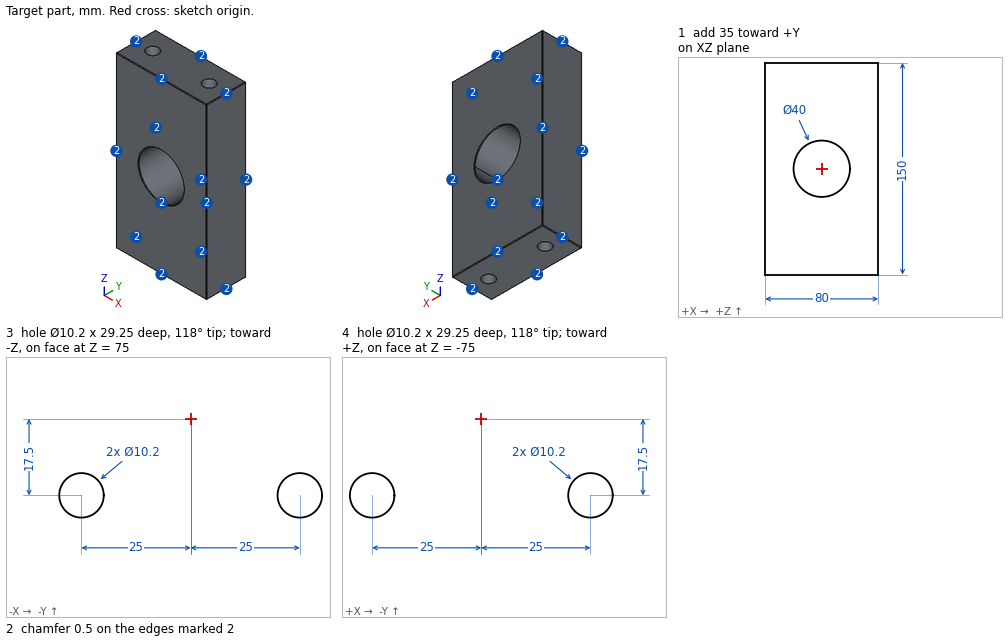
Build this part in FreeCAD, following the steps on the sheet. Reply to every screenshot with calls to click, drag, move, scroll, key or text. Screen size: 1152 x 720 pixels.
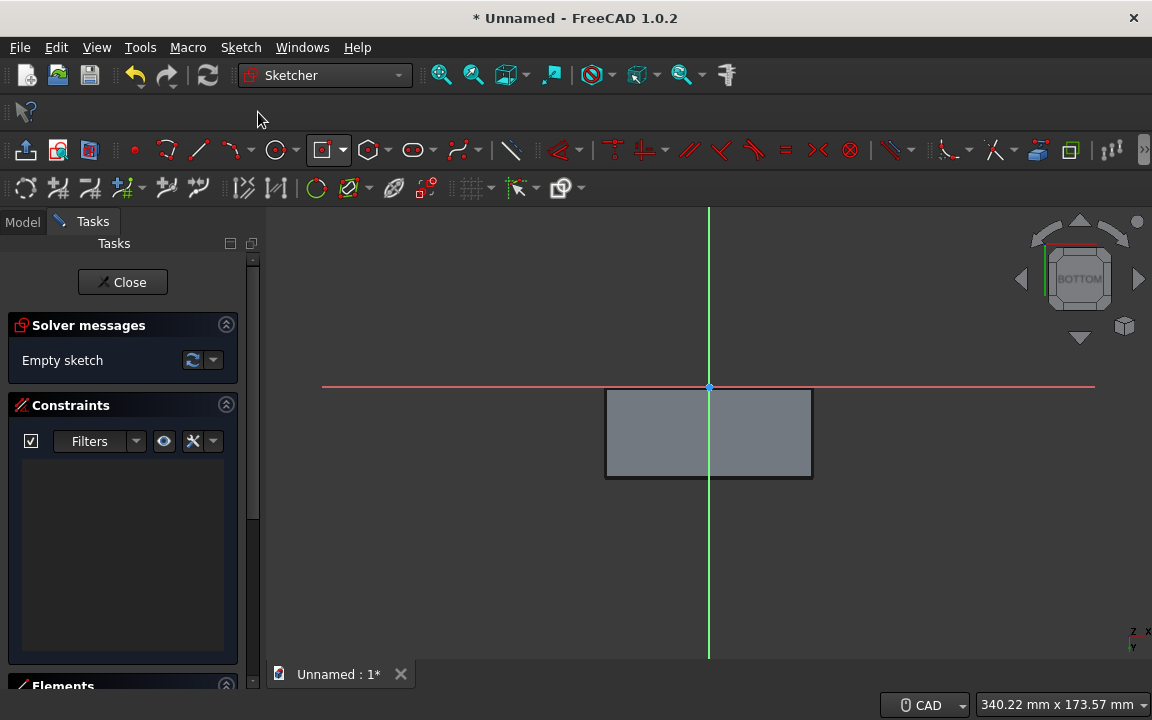
scroll(739, 410, up, 6)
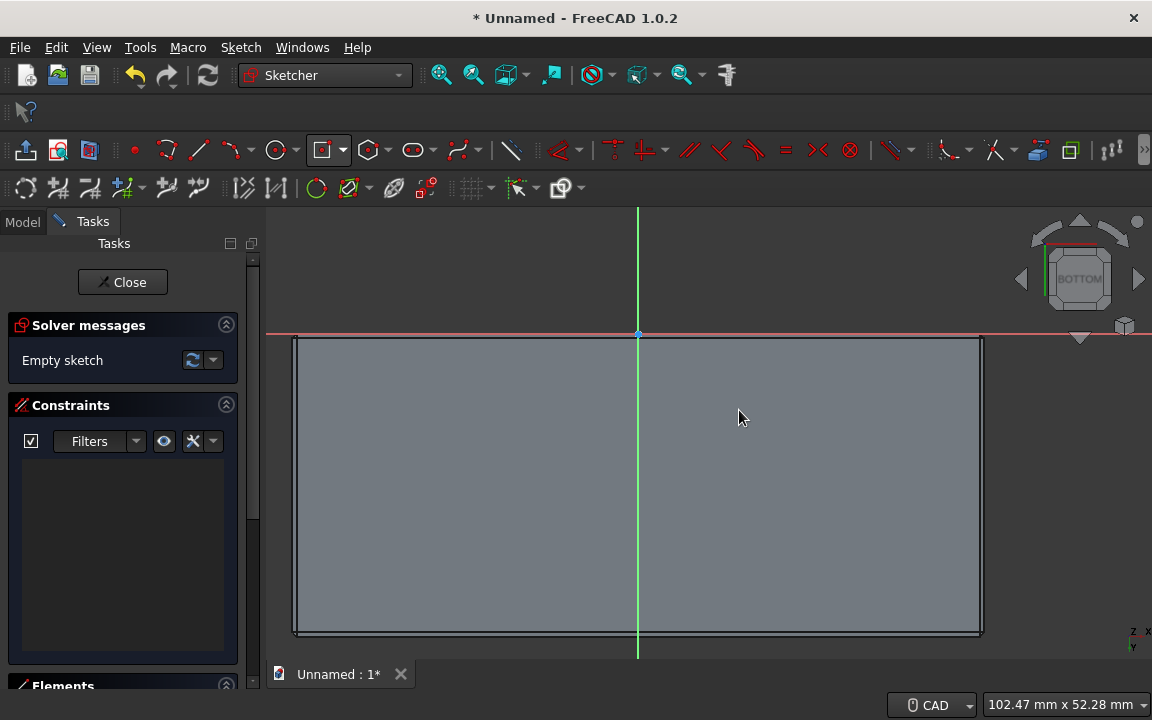
key(g)
key(c)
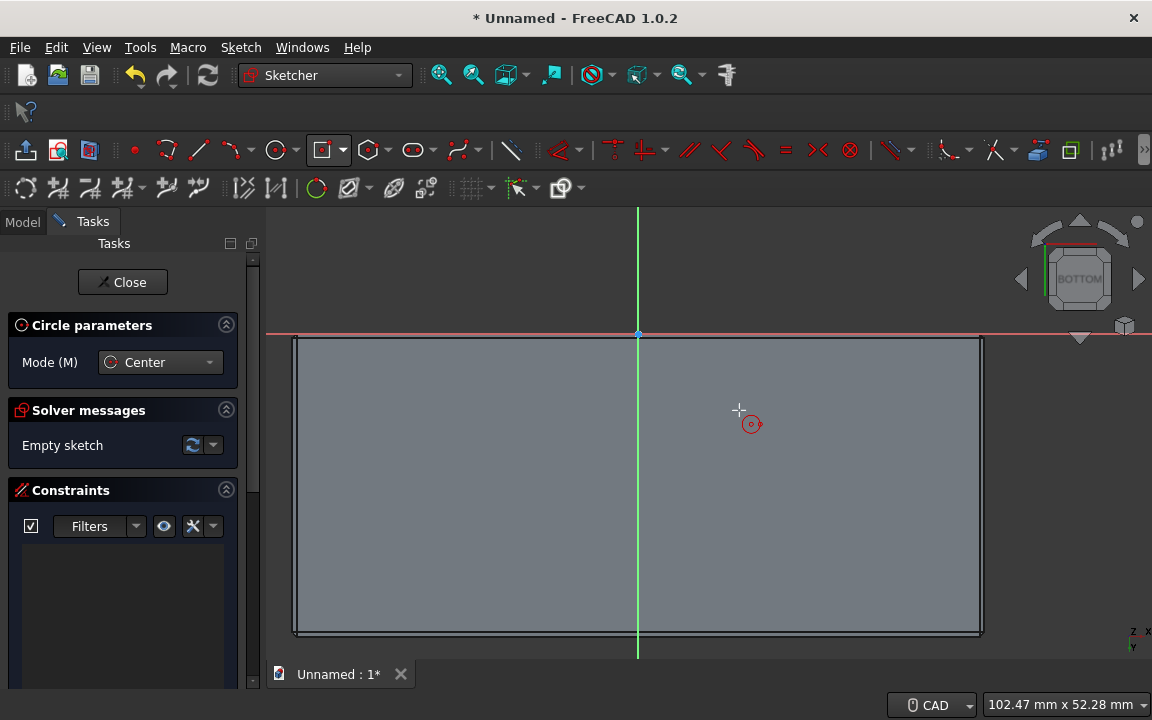
click(854, 485)
click(885, 454)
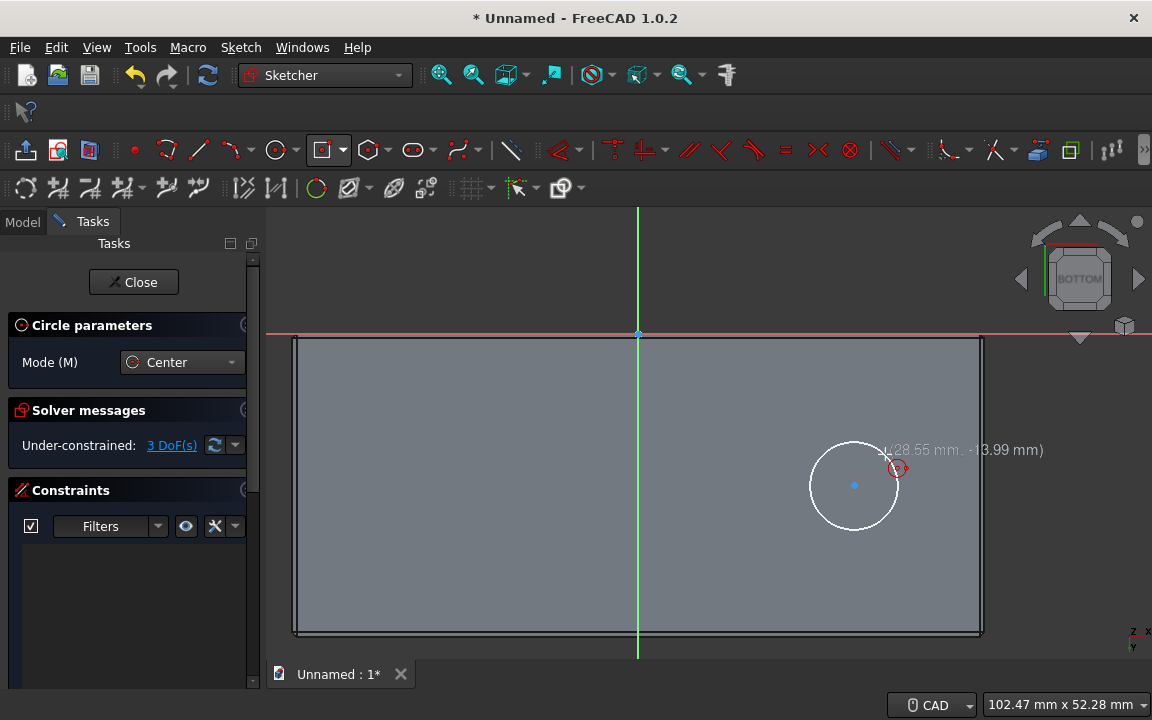
click(422, 485)
click(453, 454)
key(Escape)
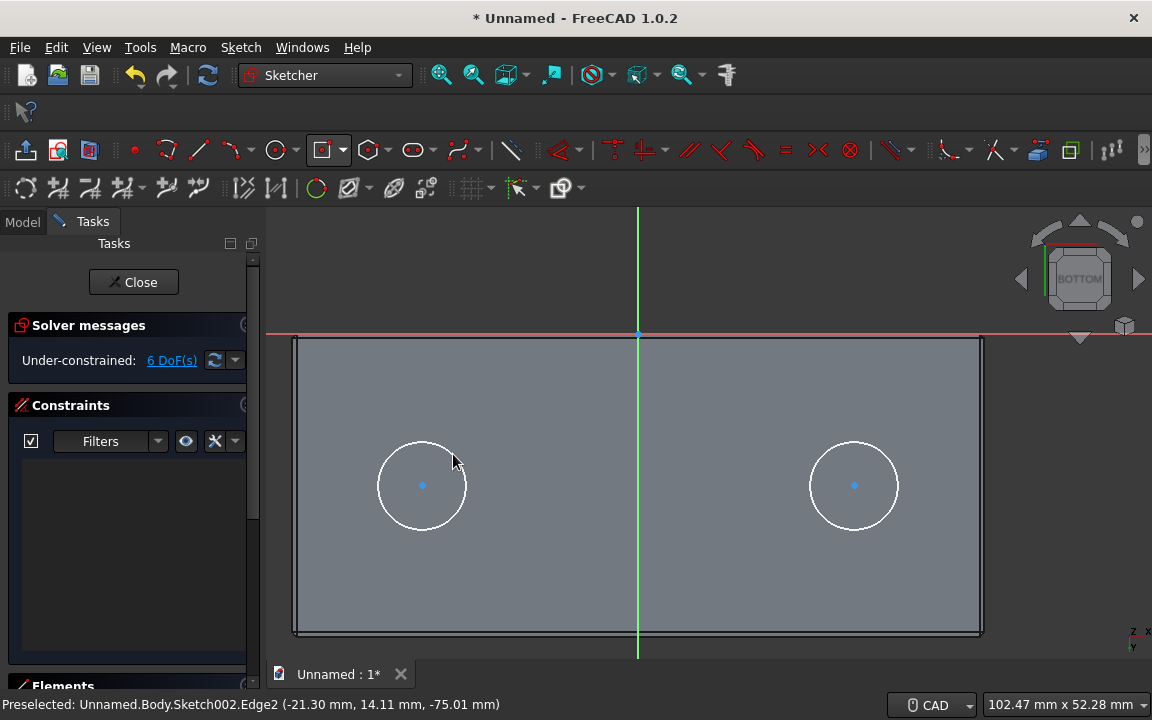
click(885, 455)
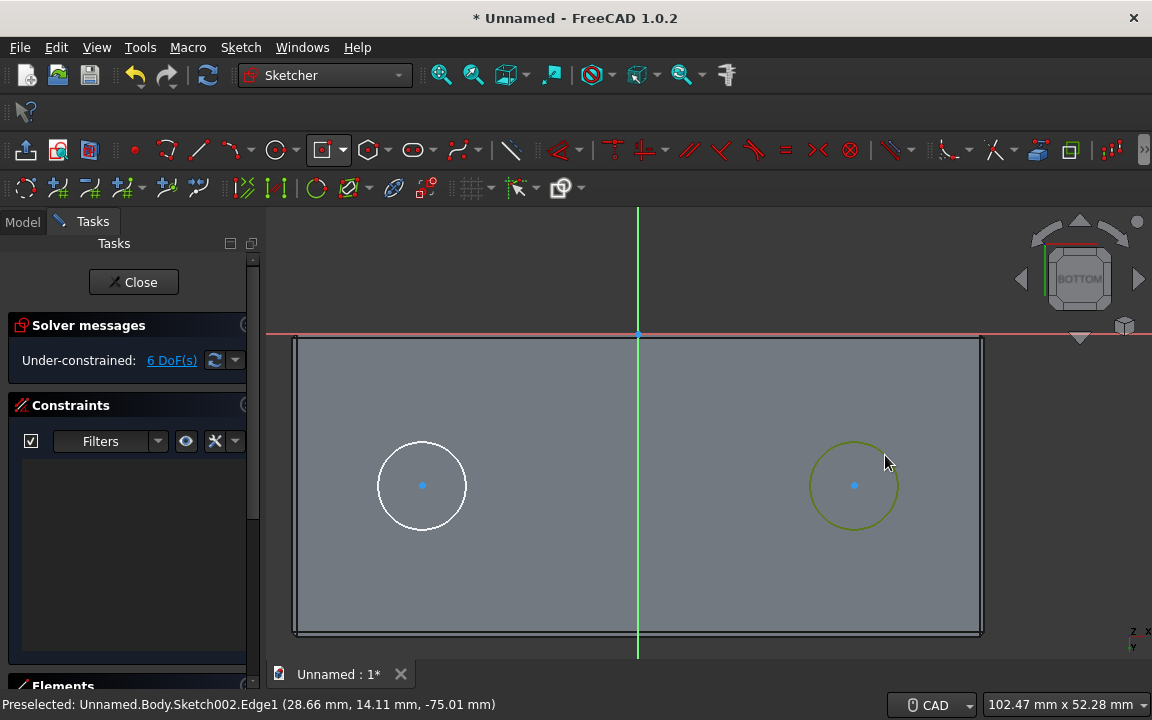
click(453, 455)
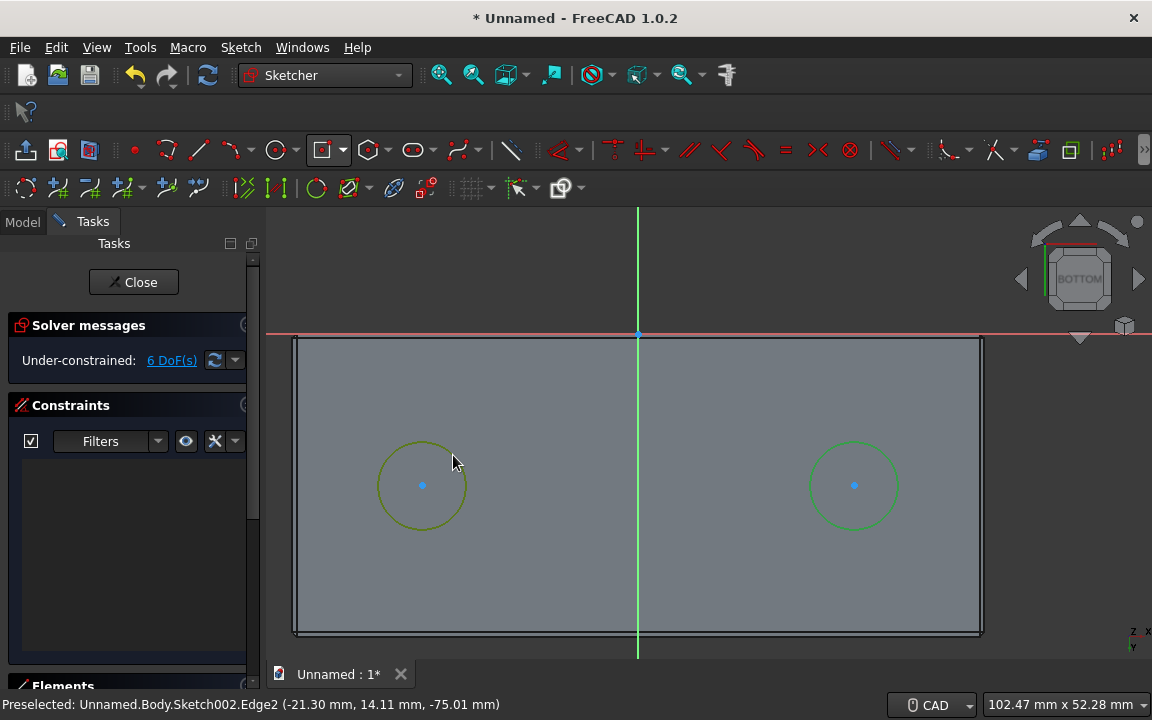
key(e)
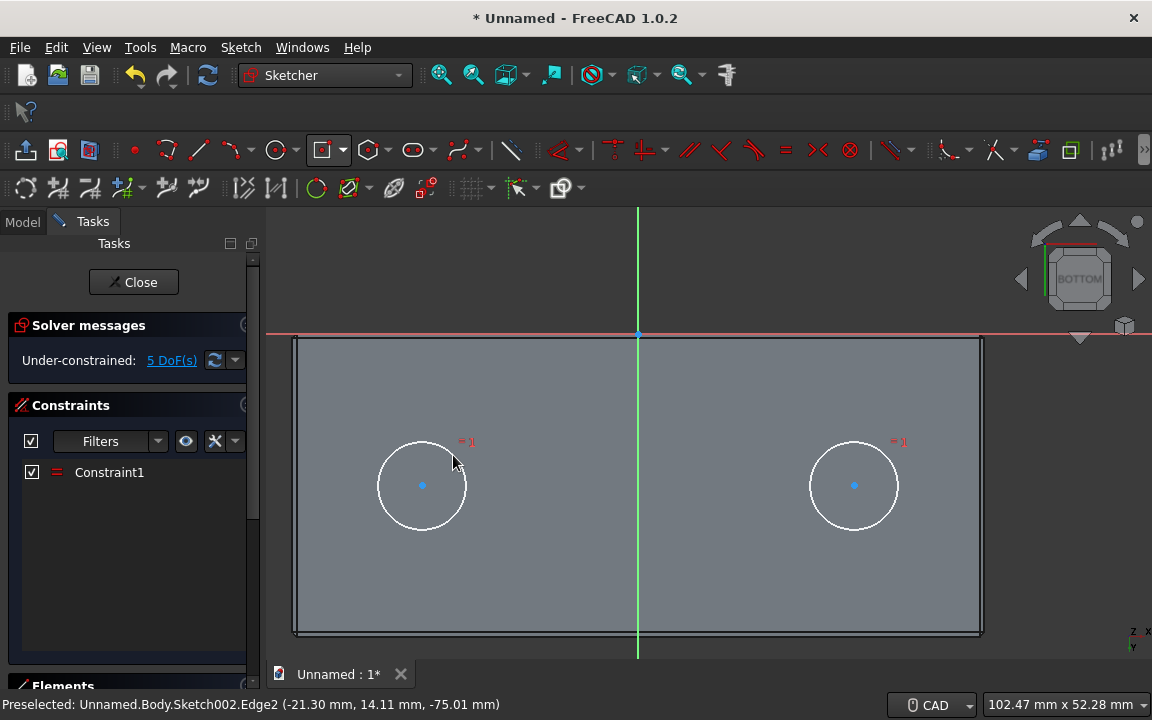
click(854, 486)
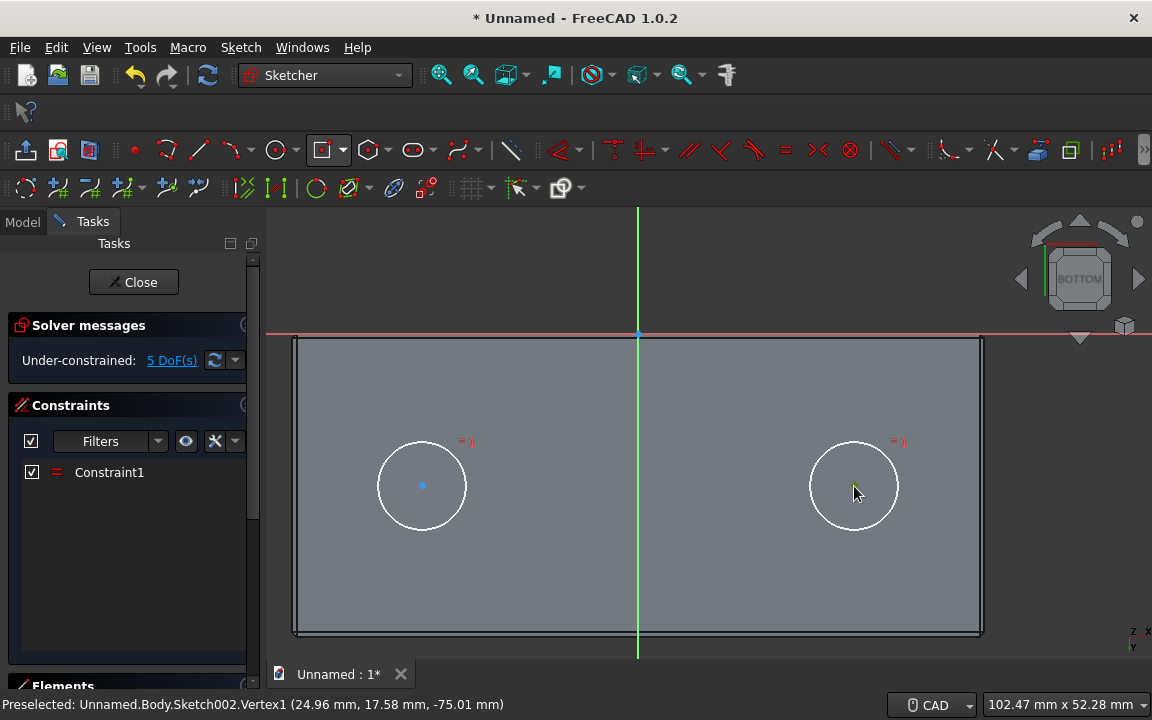
click(422, 486)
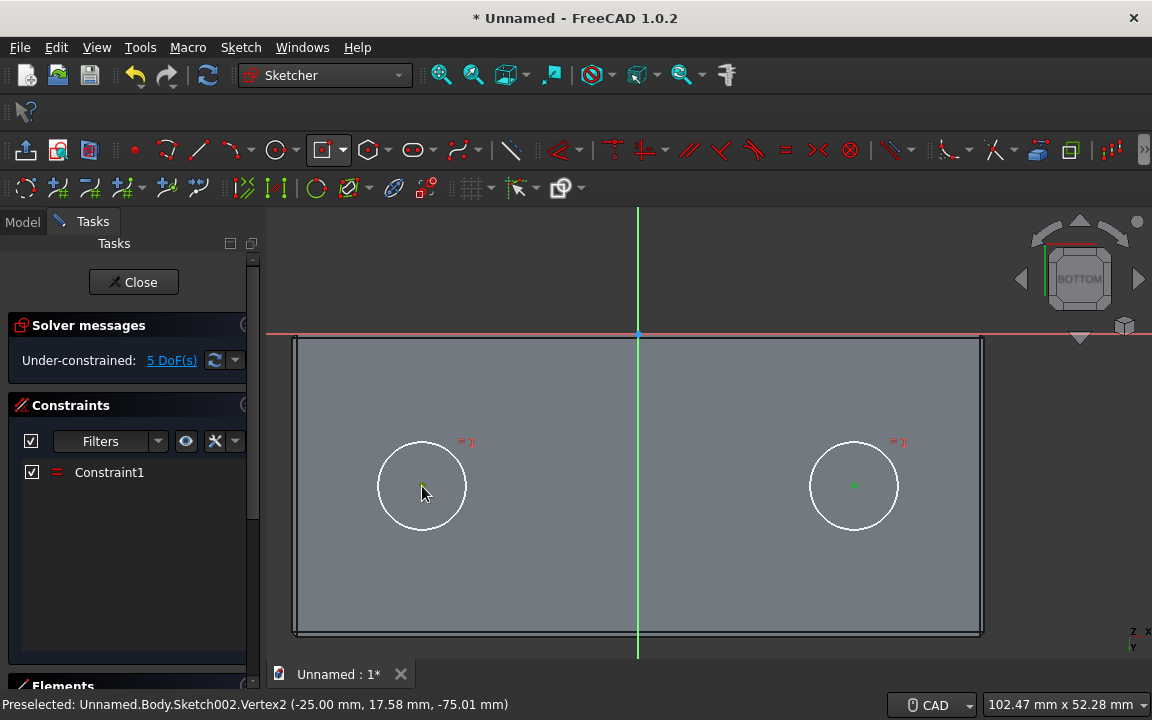
key(h)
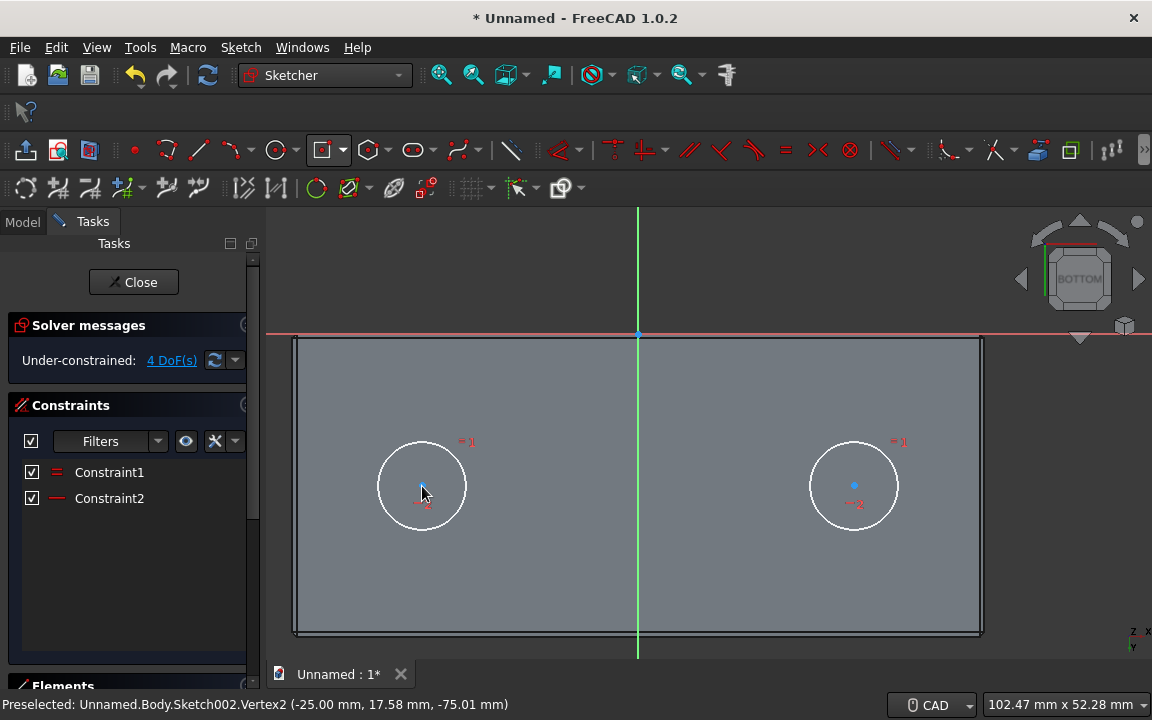
key(d)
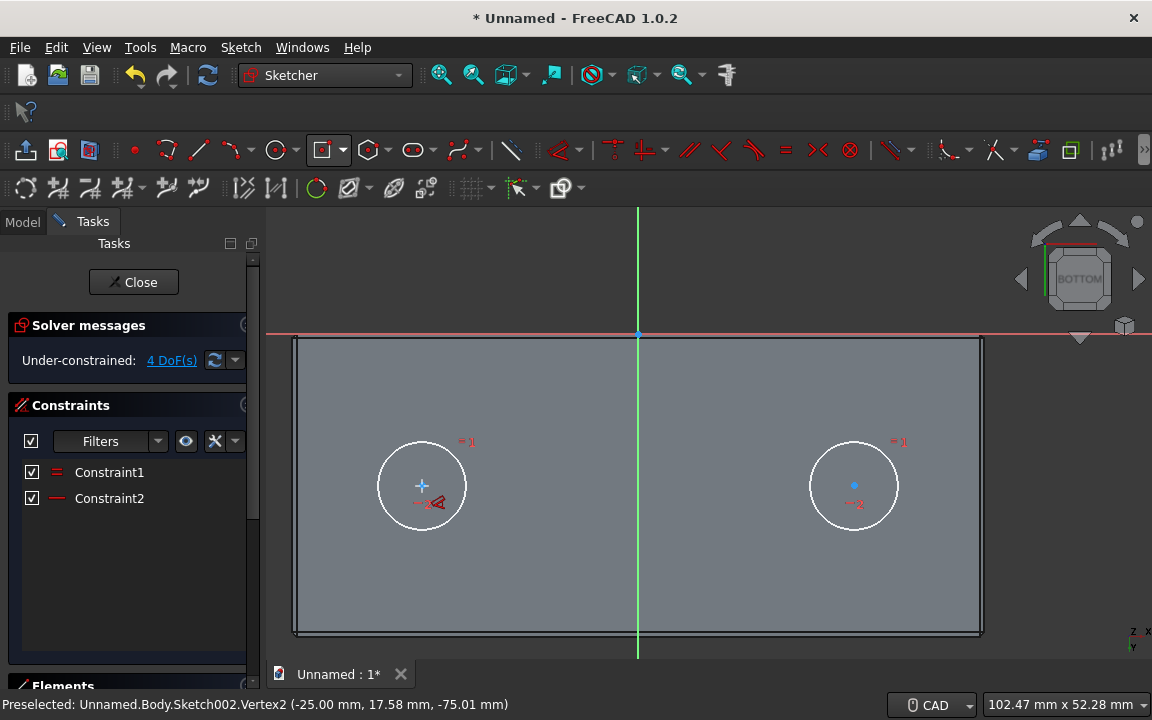
click(885, 455)
click(908, 432)